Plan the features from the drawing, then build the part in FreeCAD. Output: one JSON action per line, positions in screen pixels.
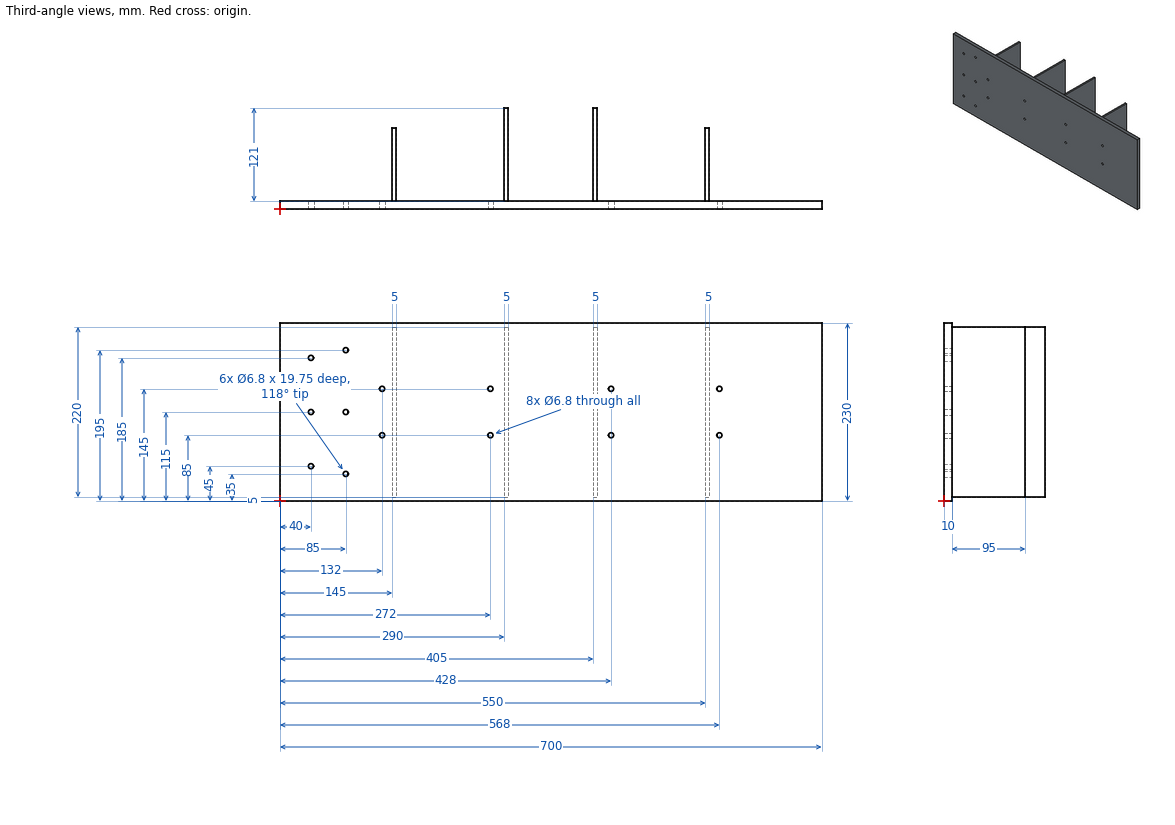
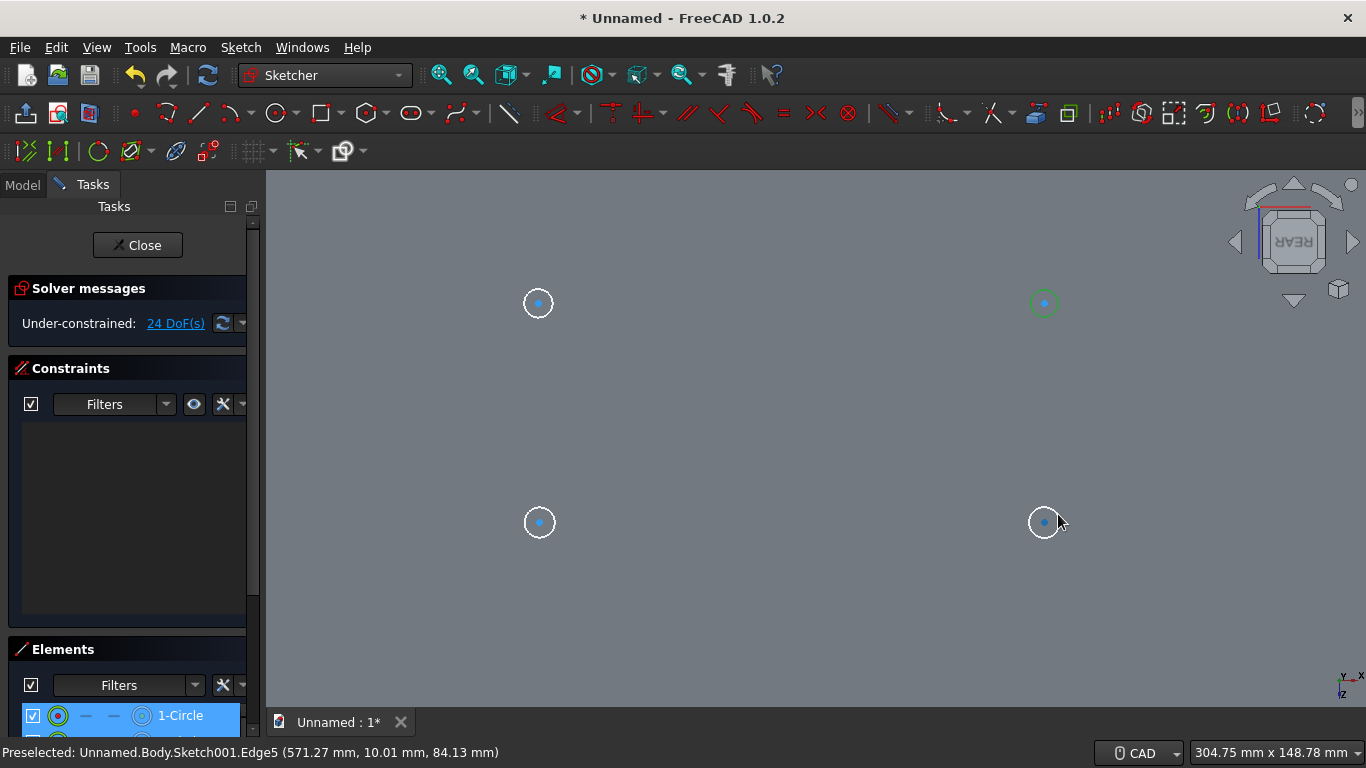
{"action": "left_click", "coordinate": [1055, 512]}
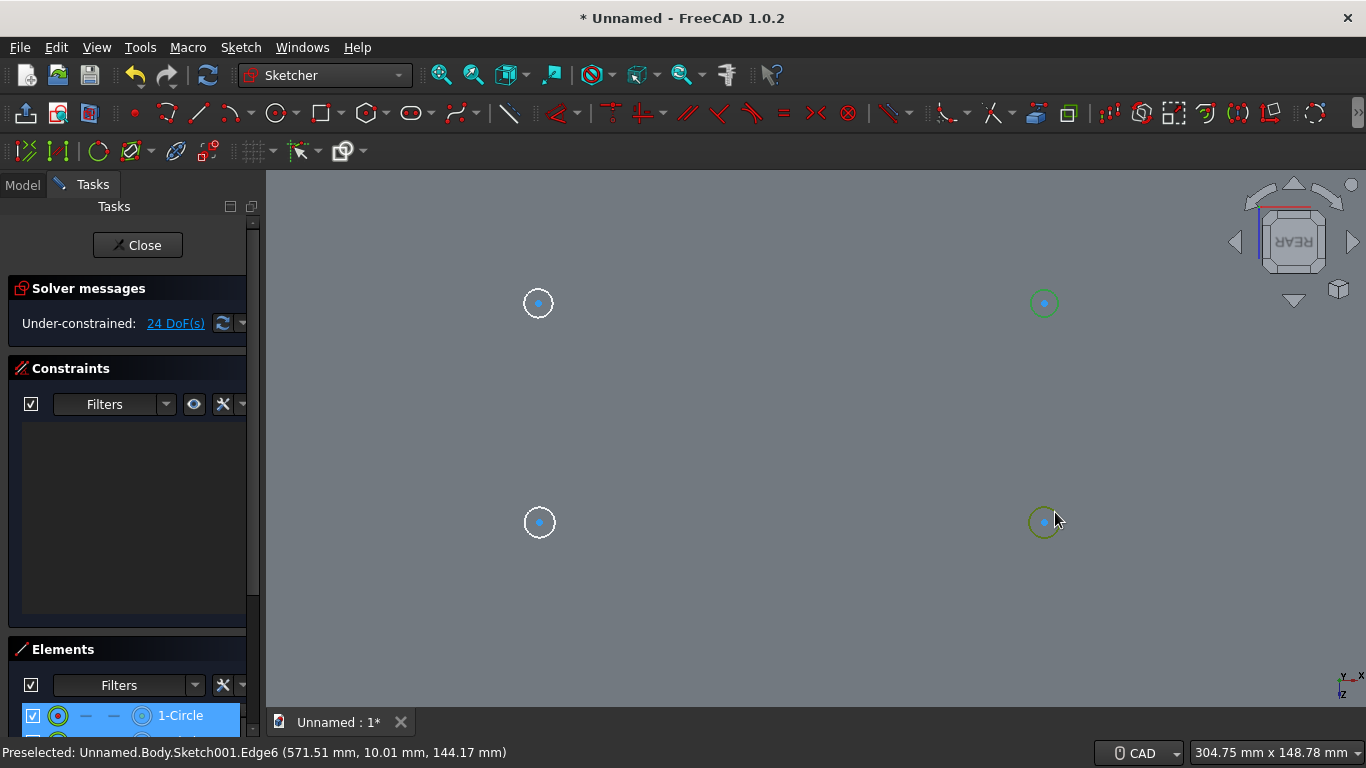
{"action": "left_click", "coordinate": [550, 512]}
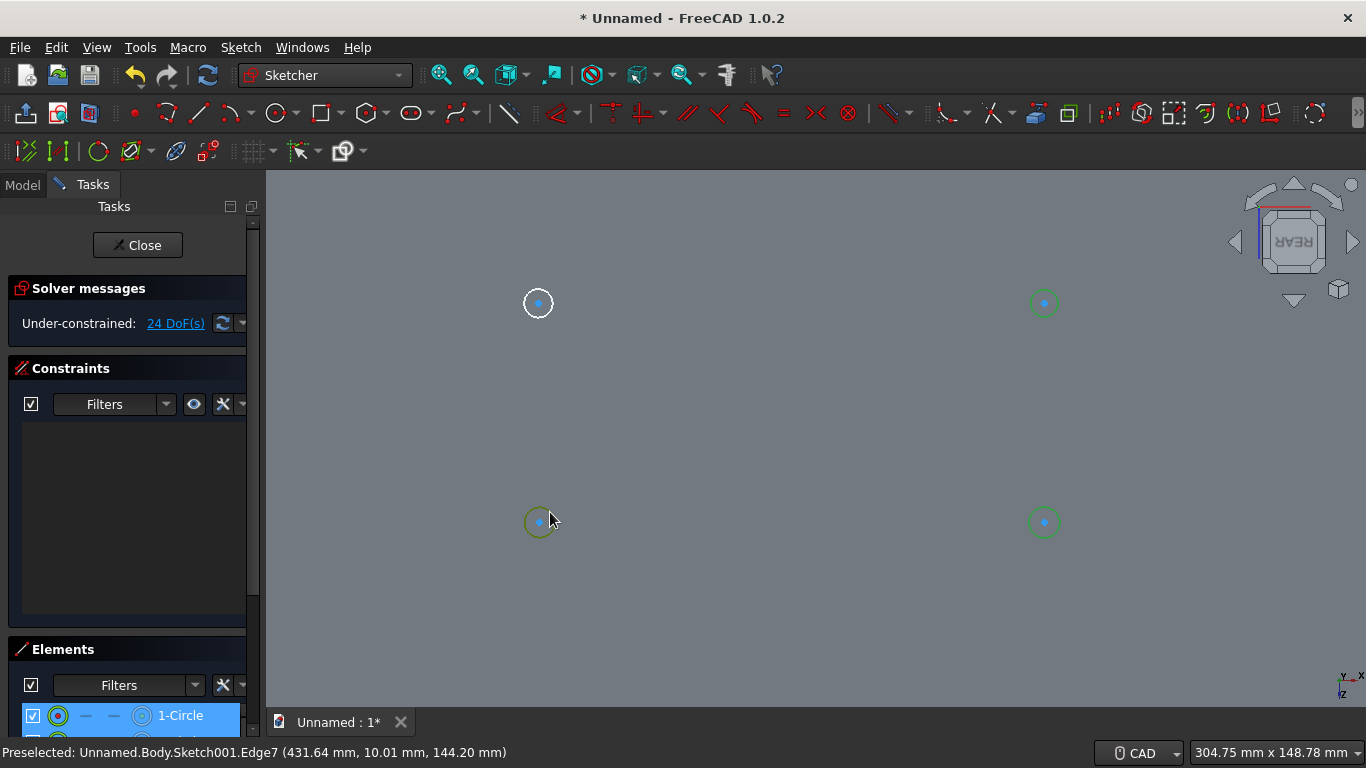
{"action": "left_click", "coordinate": [548, 293]}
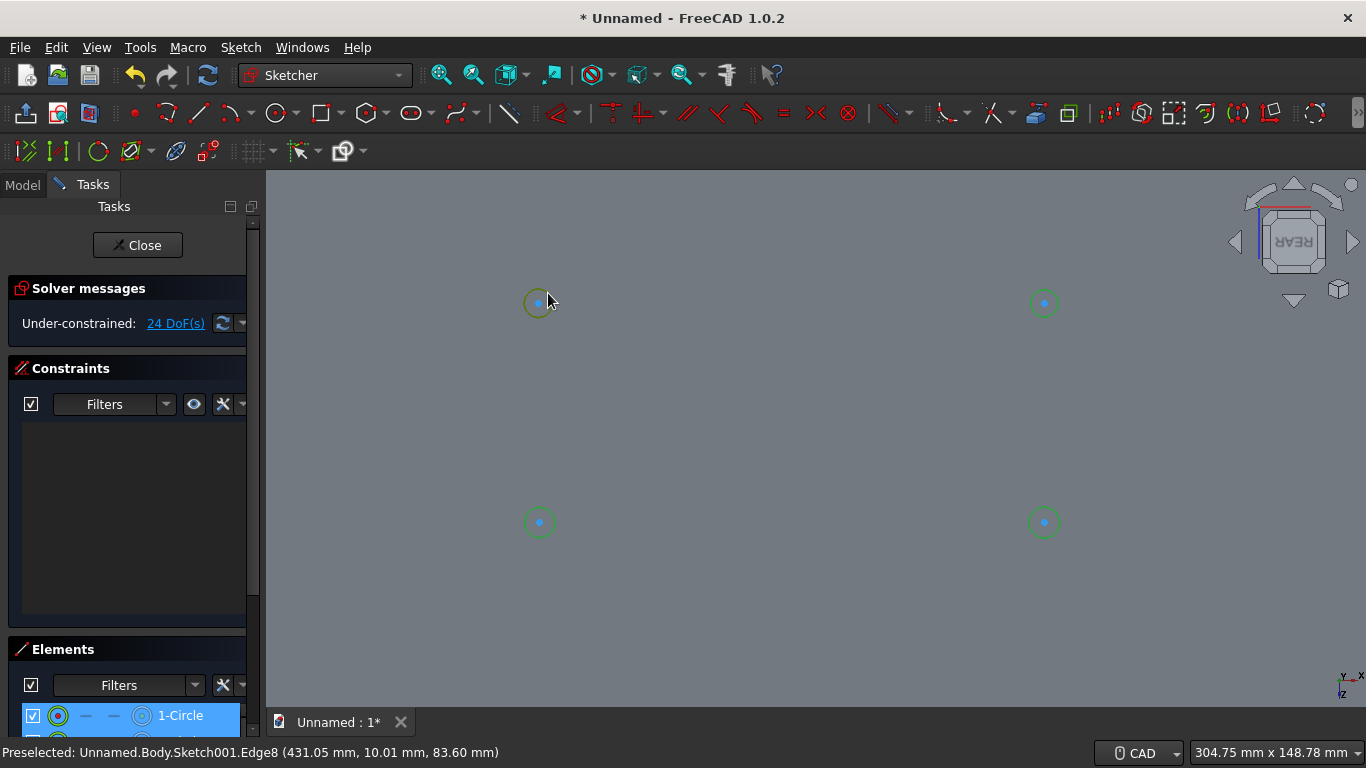
{"action": "left_click", "coordinate": [784, 114]}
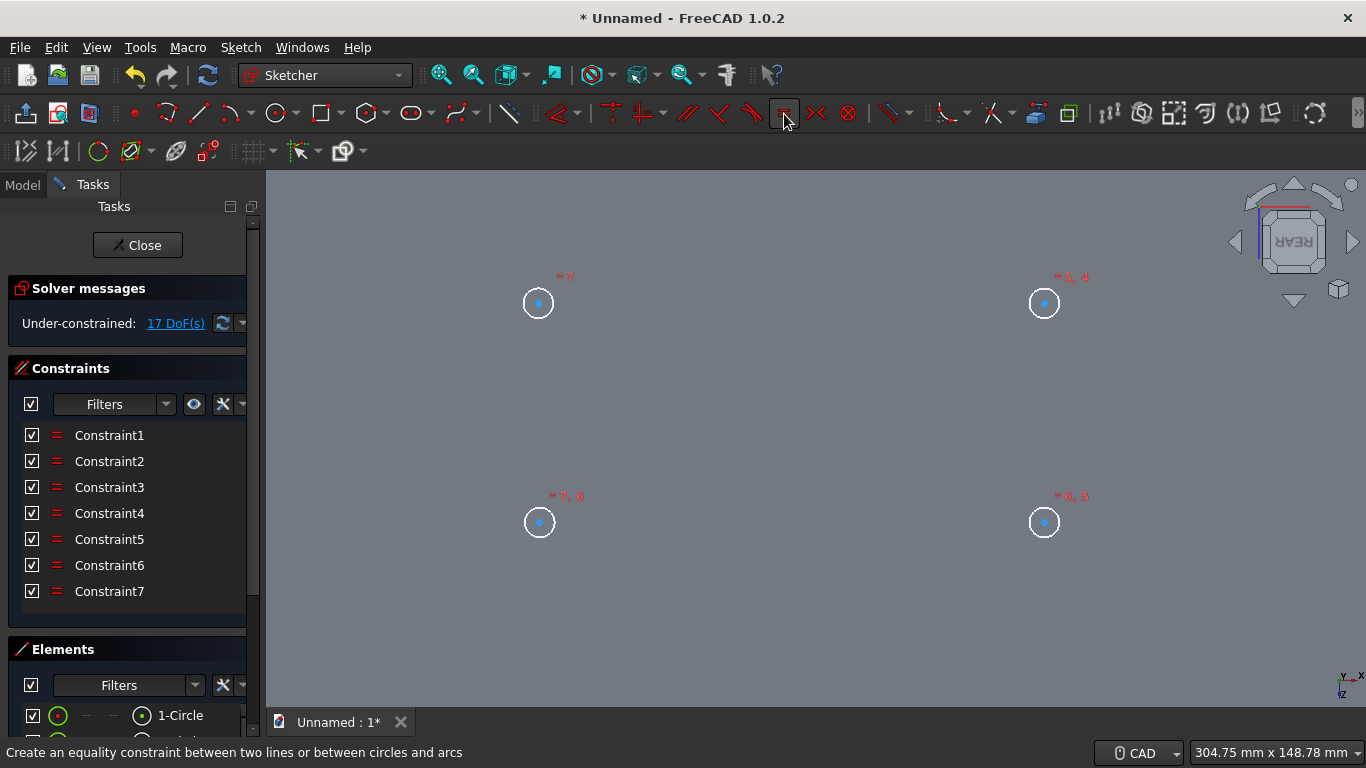
{"action": "left_click", "coordinate": [556, 114]}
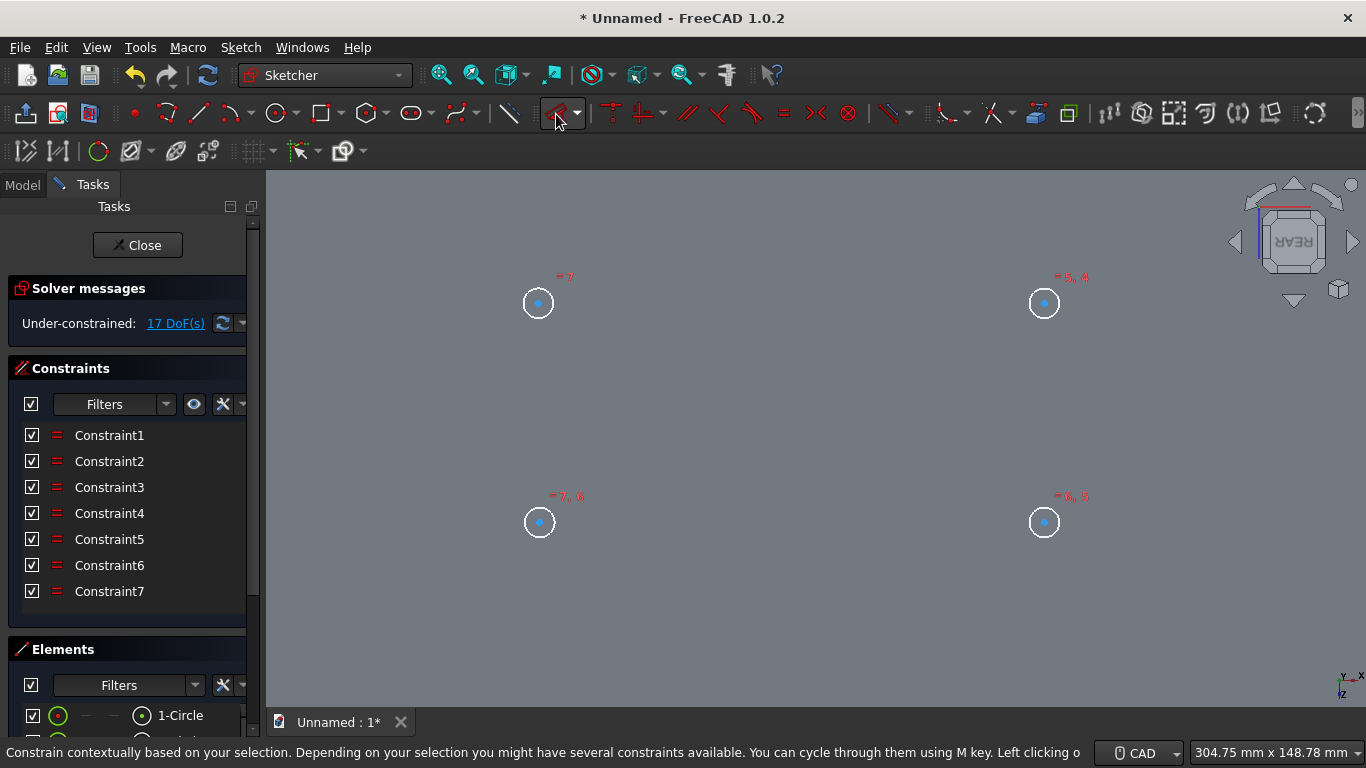
{"action": "scroll", "coordinate": [1058, 514], "scroll_direction": "down", "scroll_amount": 6}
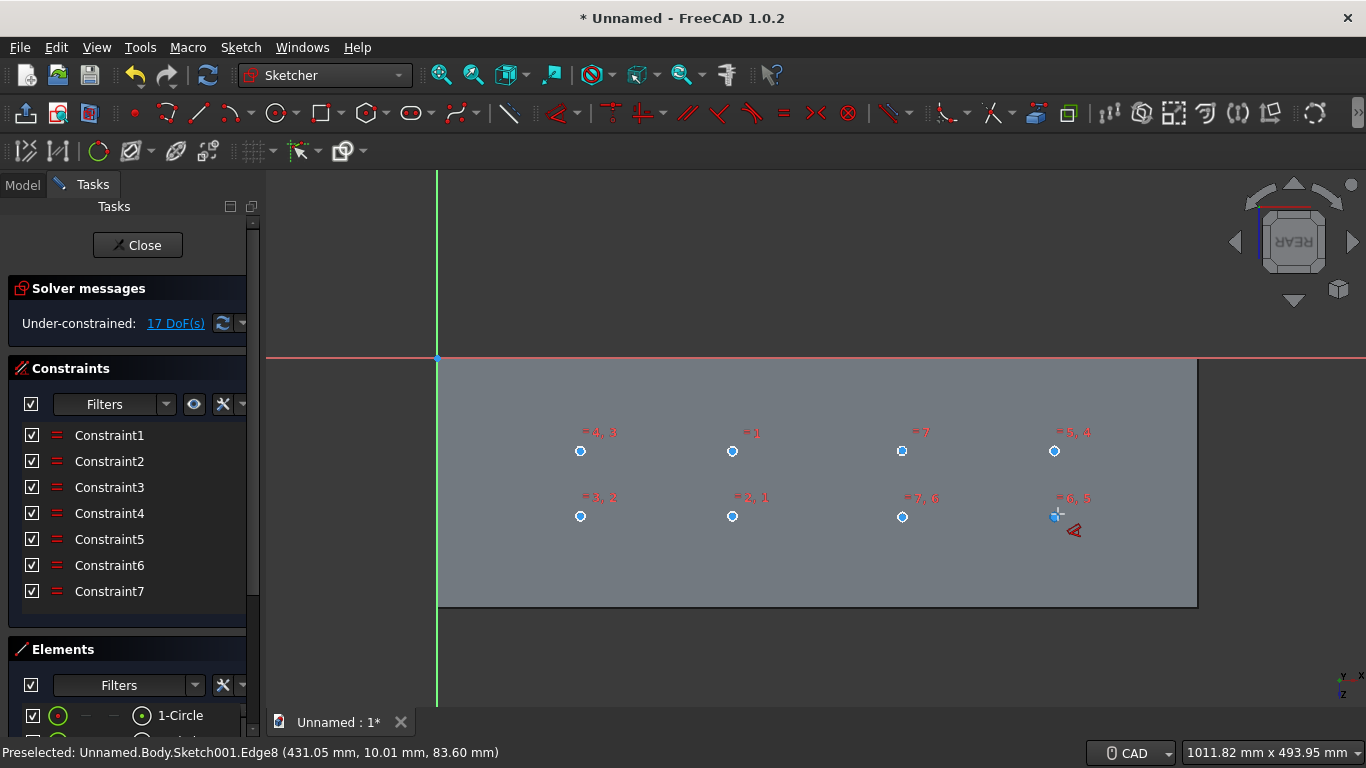
{"action": "scroll", "coordinate": [736, 448], "scroll_direction": "up", "scroll_amount": 9}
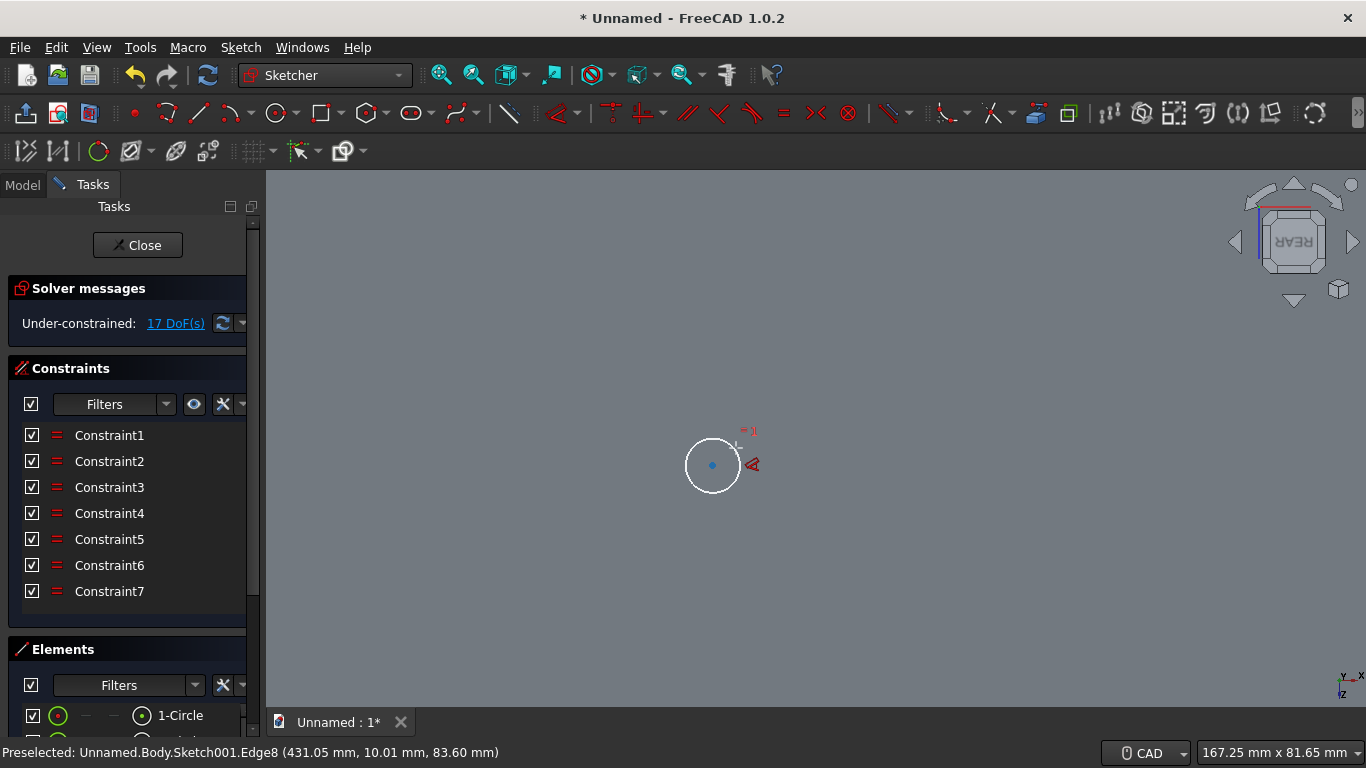
{"action": "left_click", "coordinate": [732, 447]}
{"action": "left_click", "coordinate": [755, 425]}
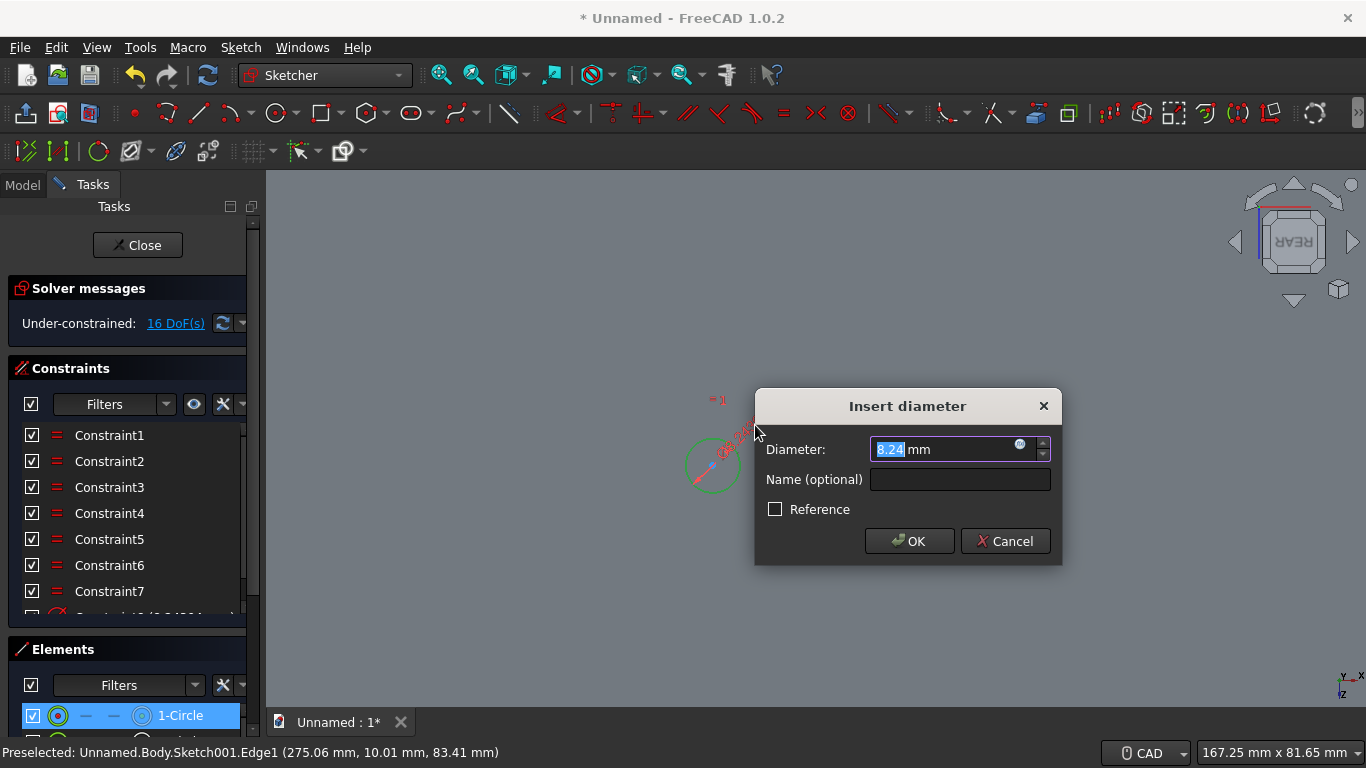
{"action": "type", "text": "6.8"}
{"action": "key", "text": "Return"}